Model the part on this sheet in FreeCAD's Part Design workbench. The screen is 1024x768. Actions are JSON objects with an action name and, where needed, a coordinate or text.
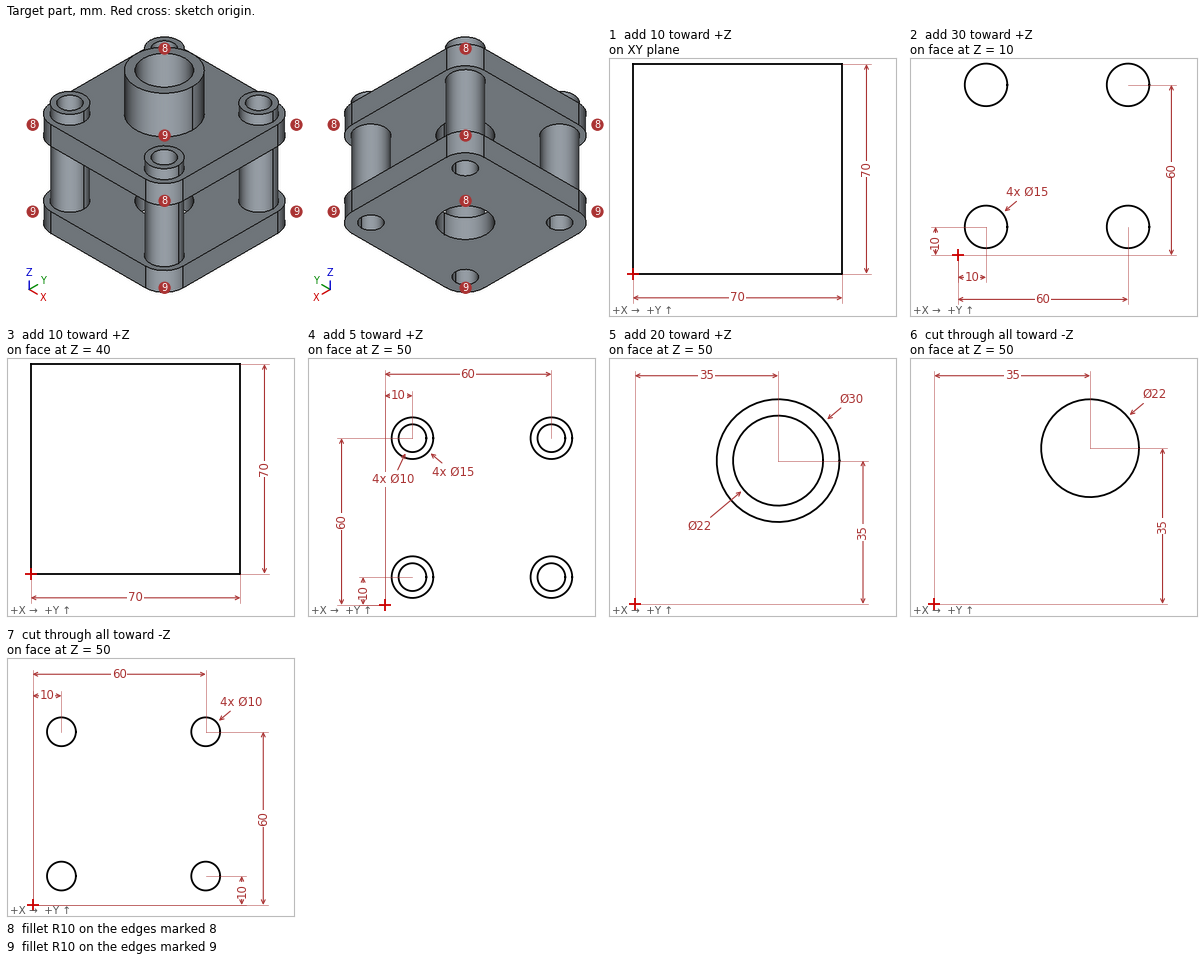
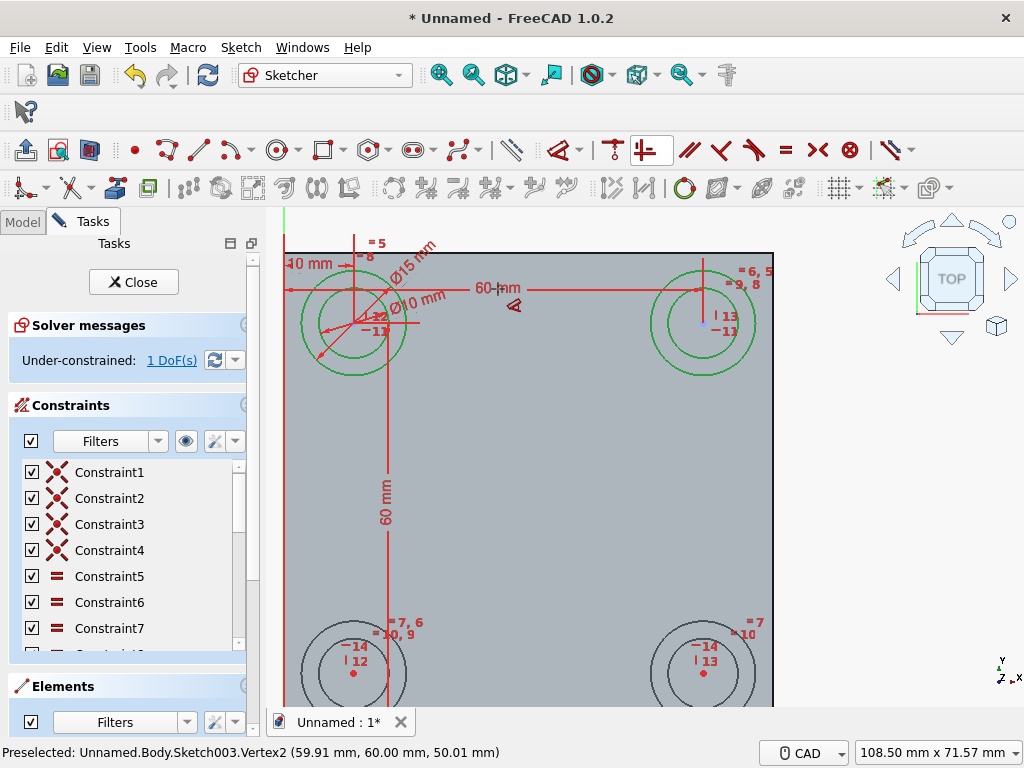
{"action": "left_click", "coordinate": [354, 674]}
{"action": "left_click", "coordinate": [436, 676]}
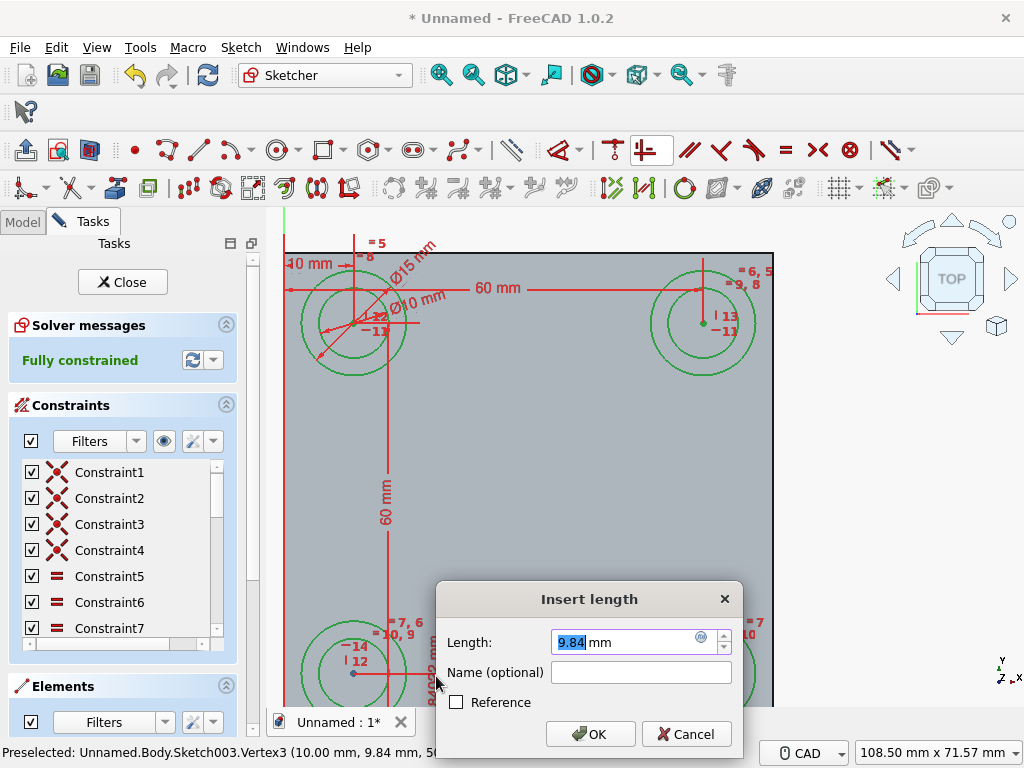
{"action": "type", "text": "10"}
{"action": "key", "text": "Return"}
{"action": "key", "text": "Escape"}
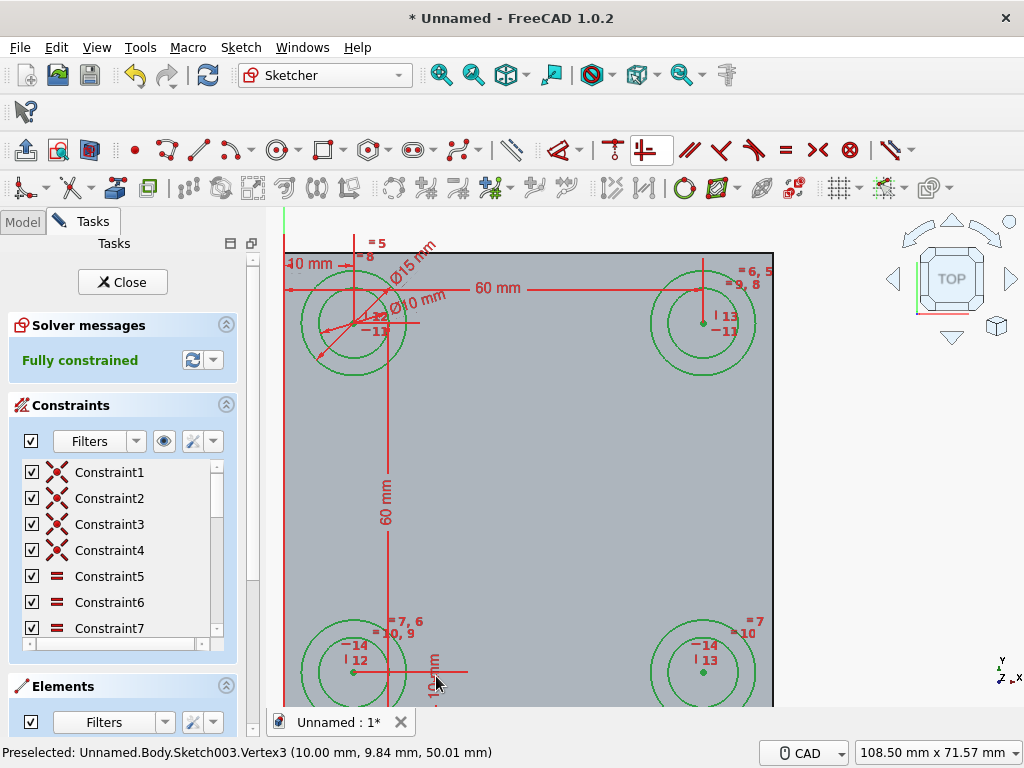
{"action": "left_click", "coordinate": [123, 282]}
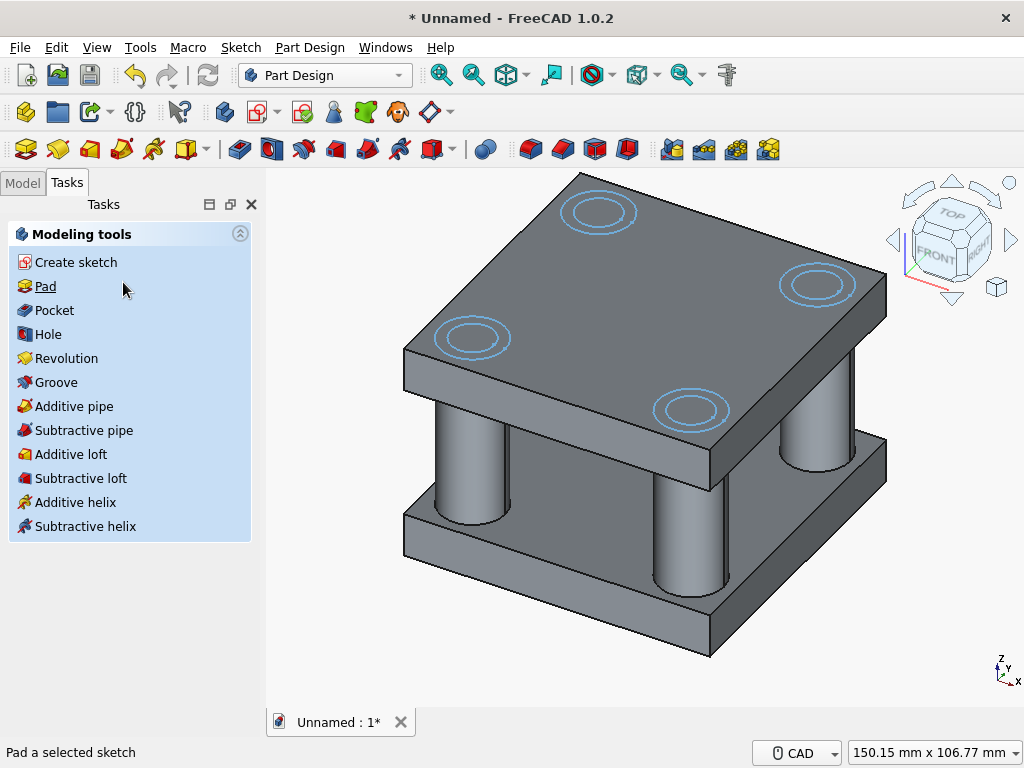
{"action": "left_click", "coordinate": [26, 150]}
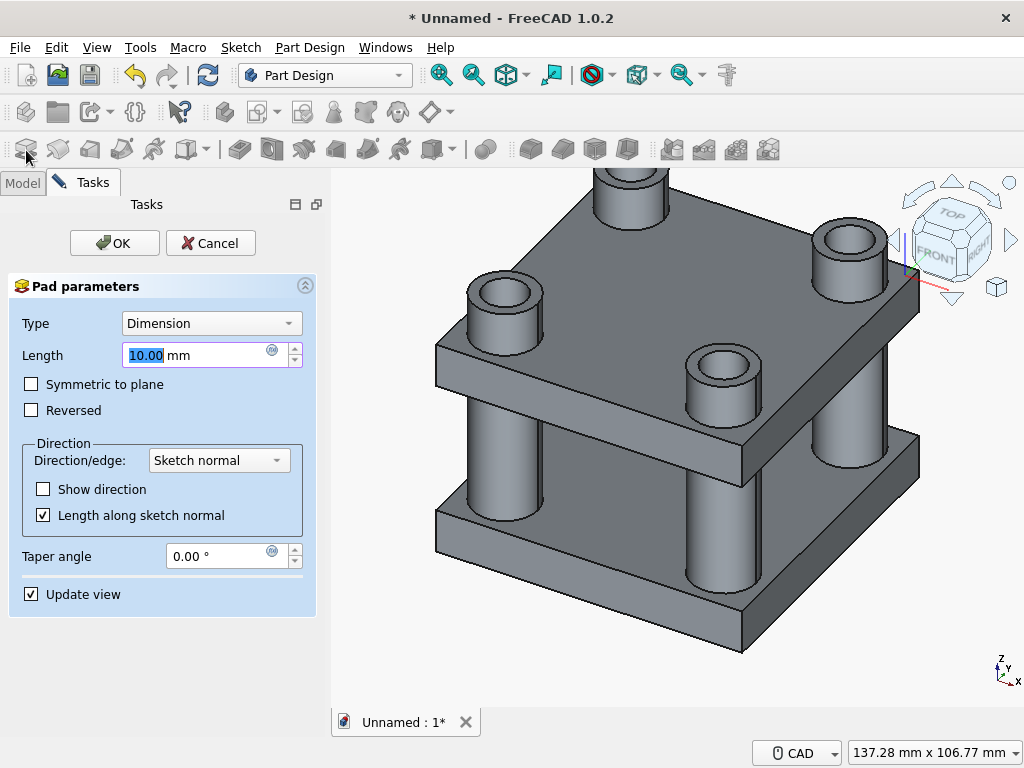
{"action": "type", "text": "5"}
{"action": "key", "text": "Tab"}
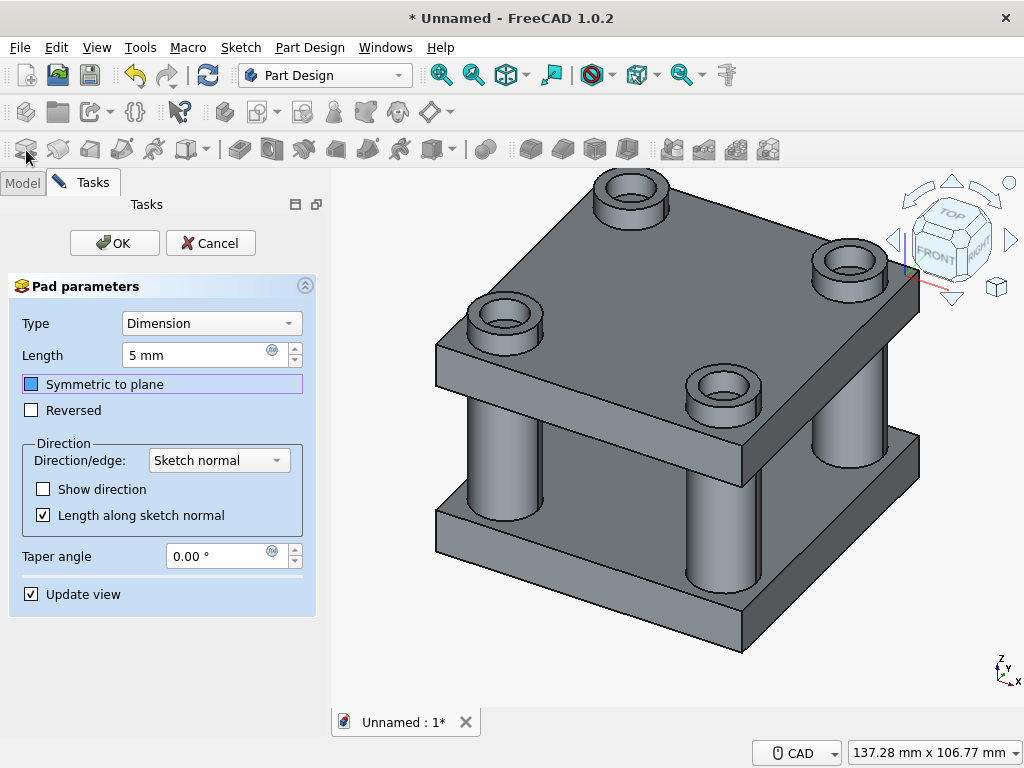
{"action": "left_click", "coordinate": [115, 243]}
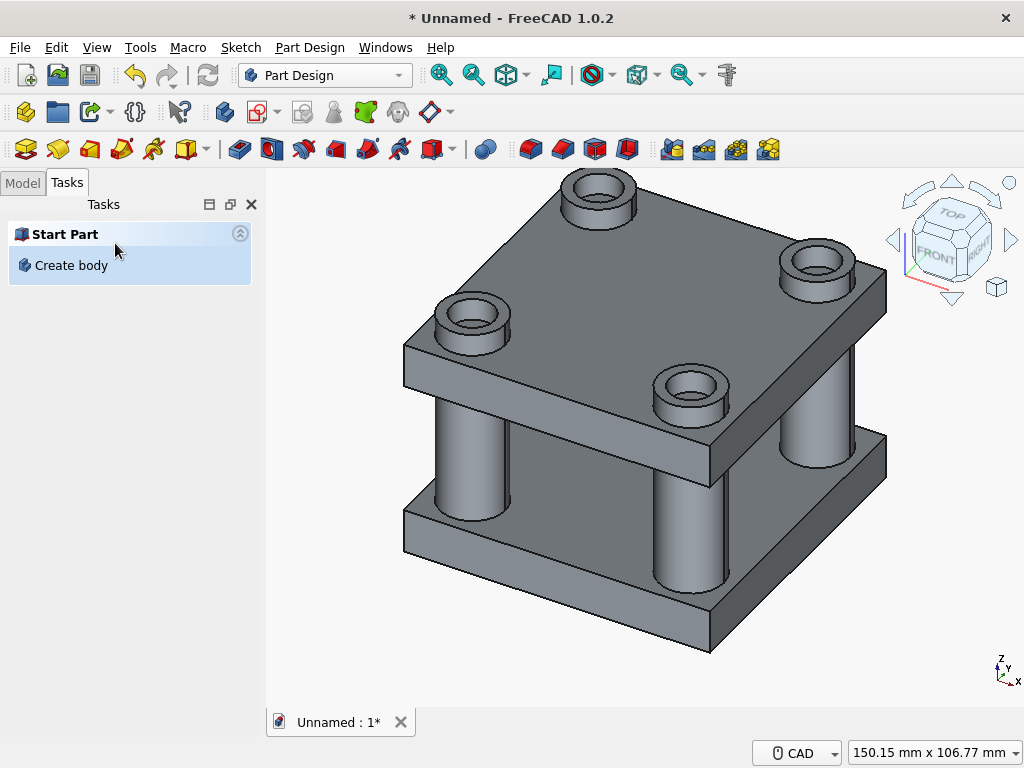
{"action": "key", "text": "v f"}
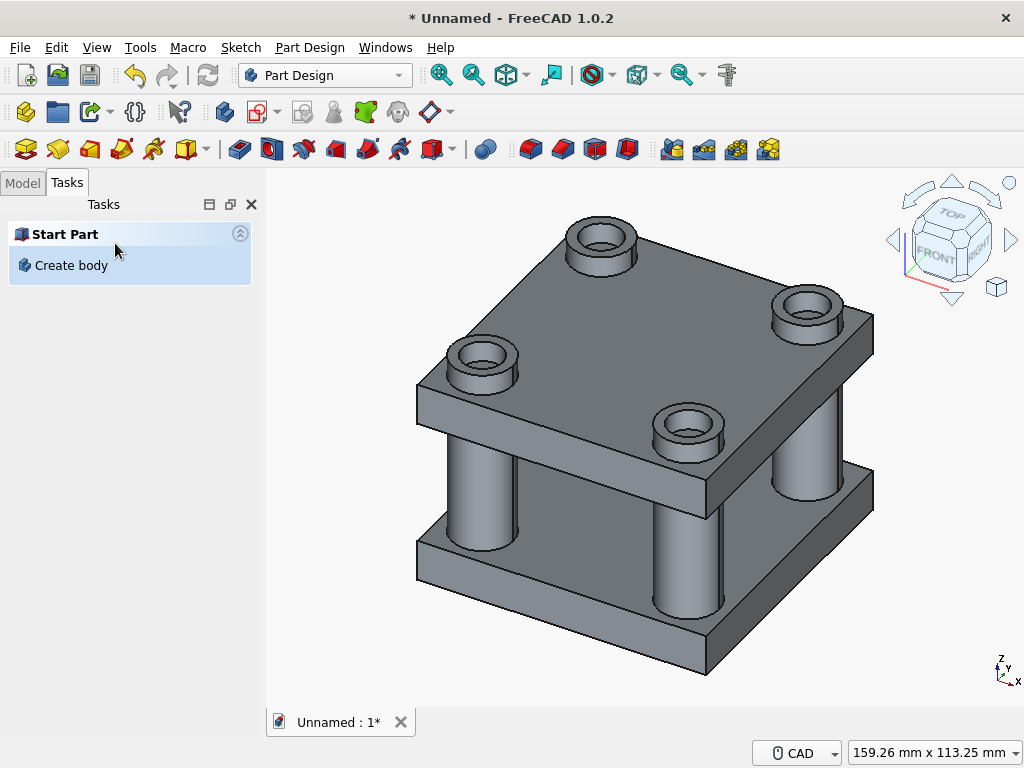
{"action": "left_click", "coordinate": [645, 349]}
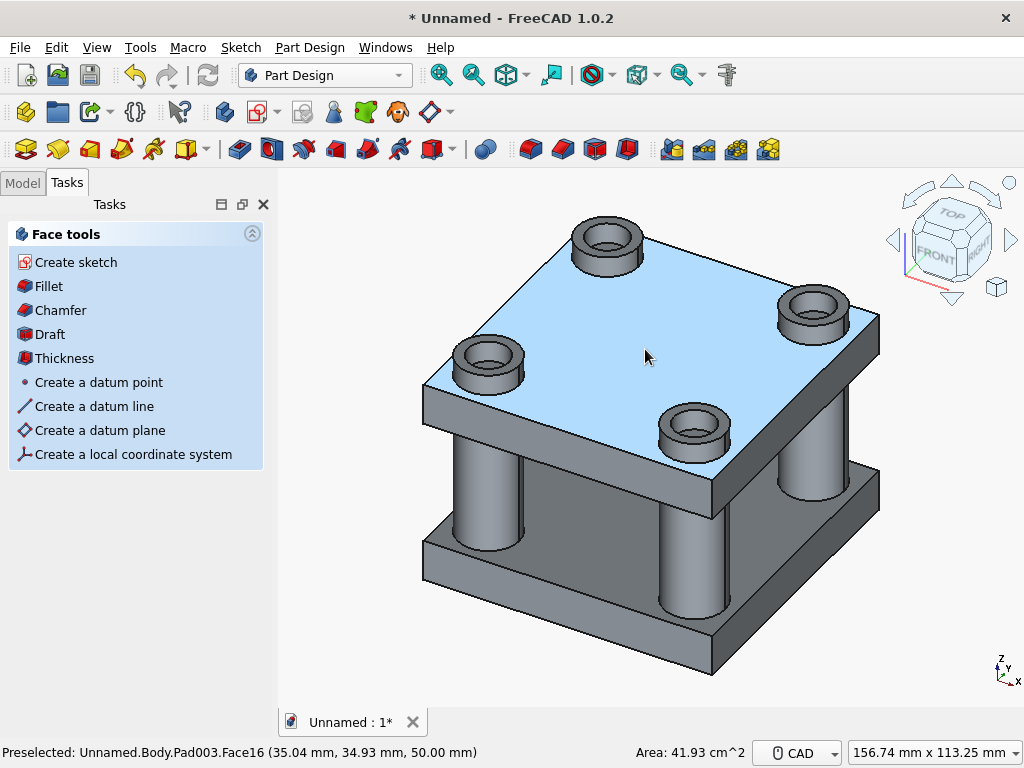
{"action": "left_click", "coordinate": [258, 112]}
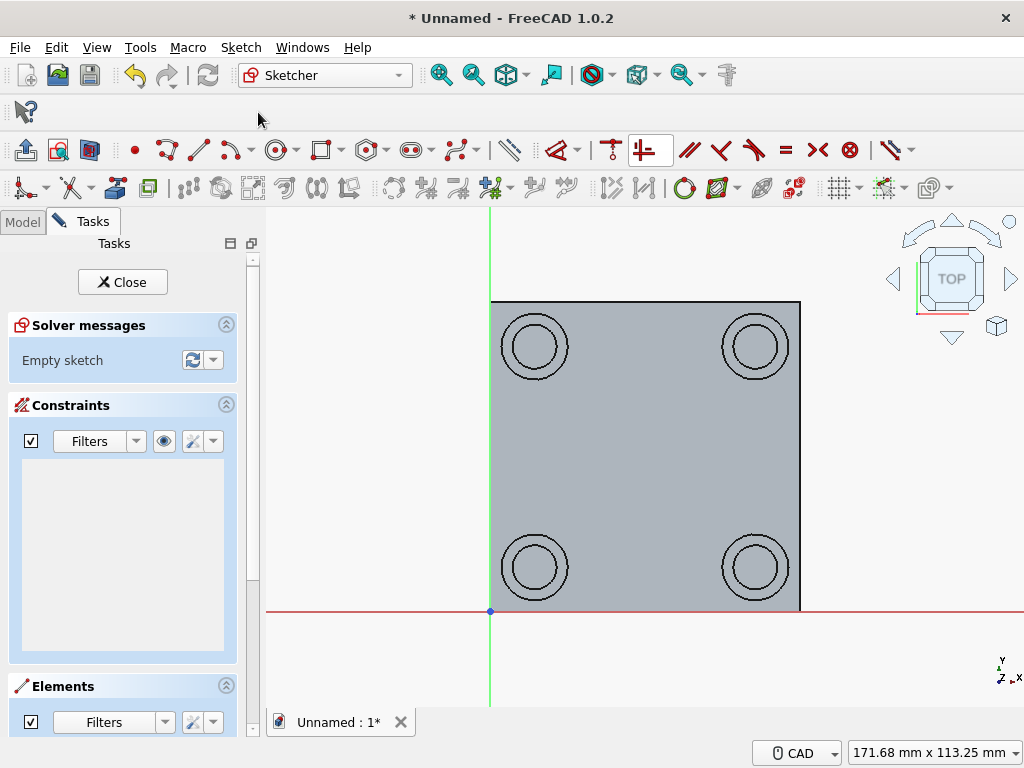
{"action": "key", "text": "q s"}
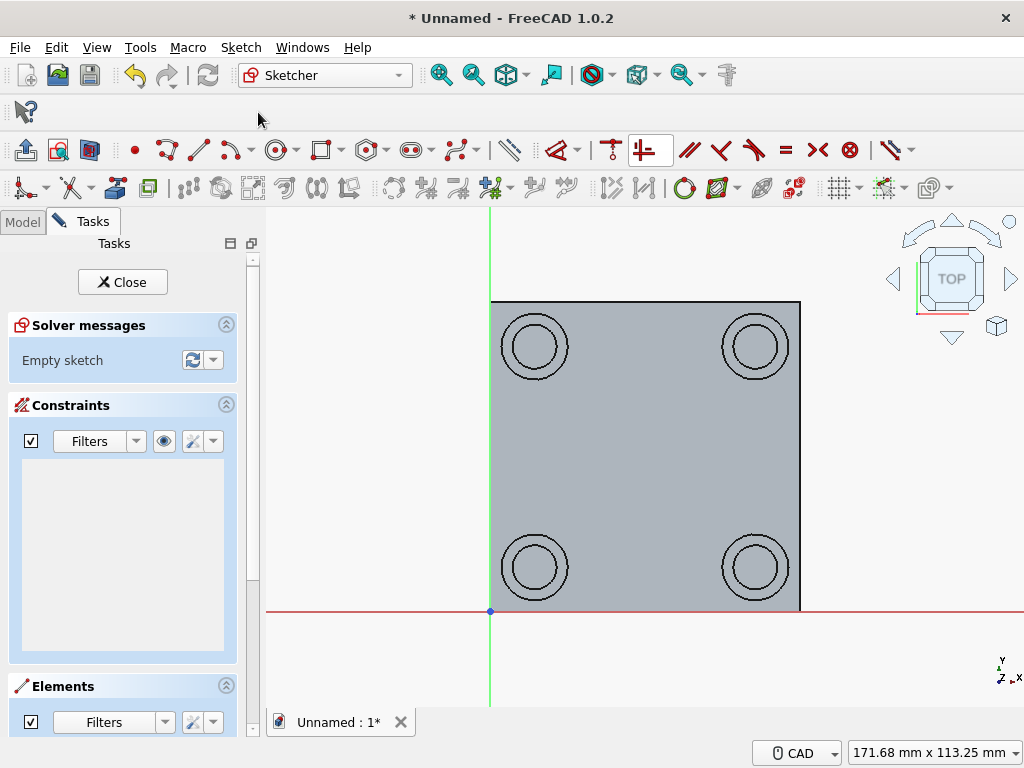
{"action": "scroll", "coordinate": [650, 591], "scroll_direction": "up", "scroll_amount": 2}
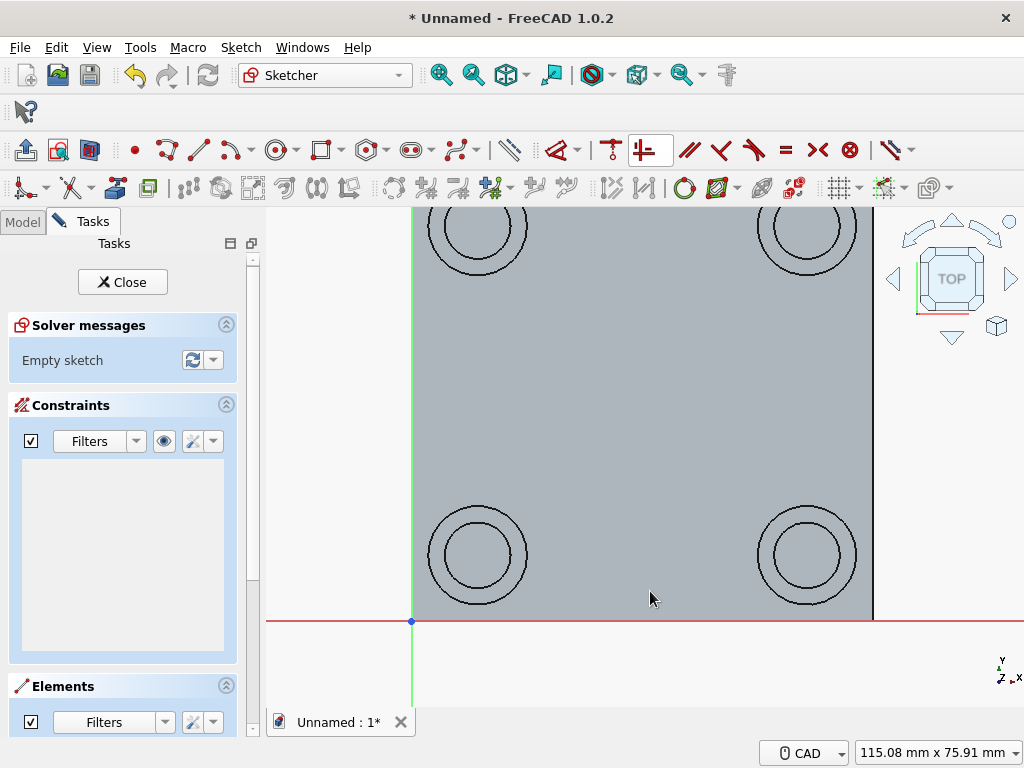
{"action": "left_click", "coordinate": [276, 150]}